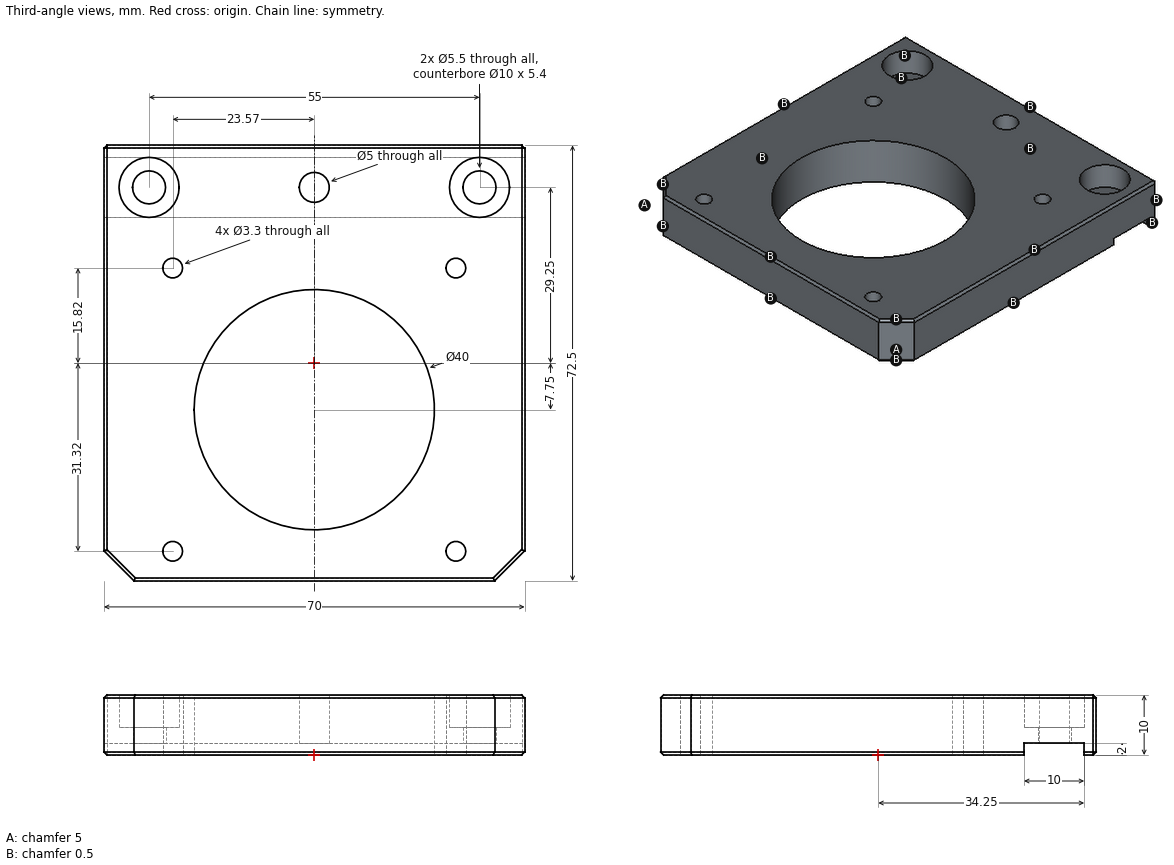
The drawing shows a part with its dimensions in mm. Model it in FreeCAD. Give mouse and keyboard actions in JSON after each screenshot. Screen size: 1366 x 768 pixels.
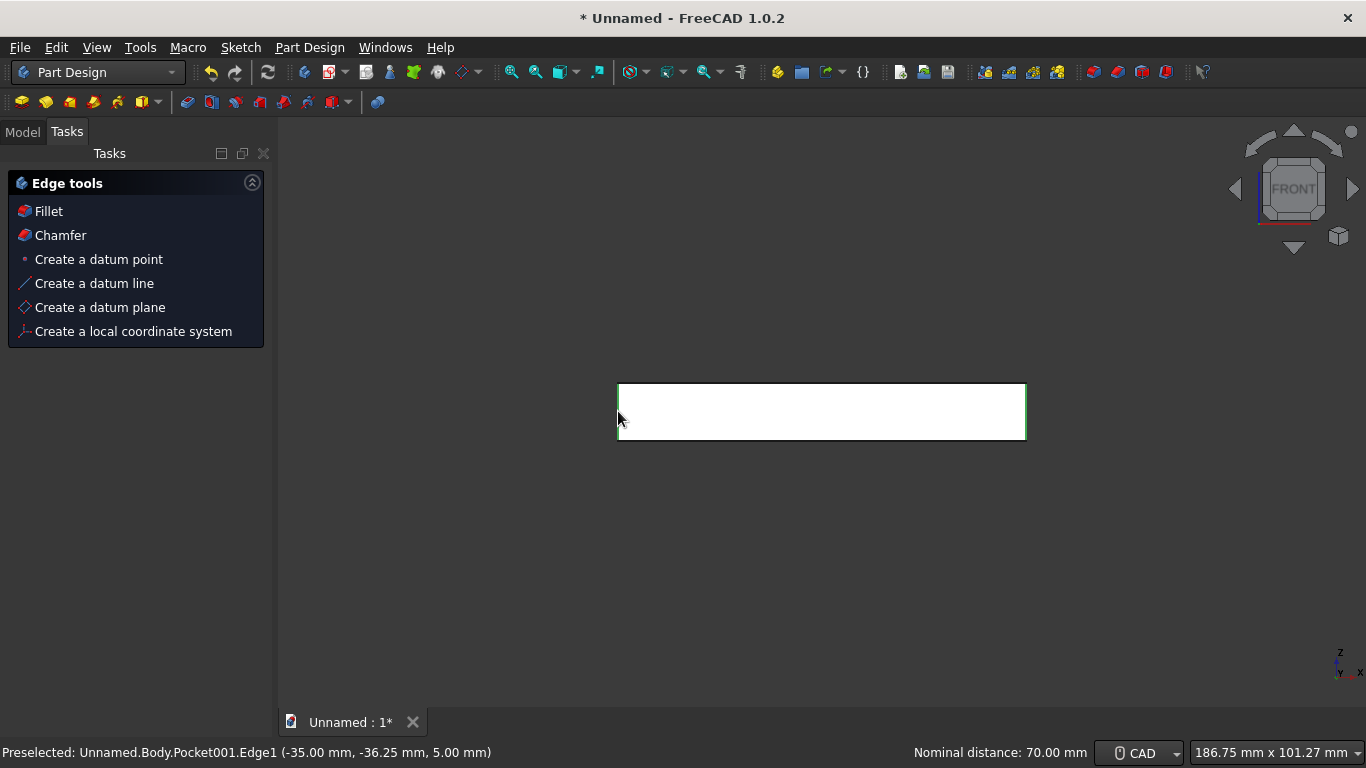
{"action": "left_click", "coordinate": [1118, 72]}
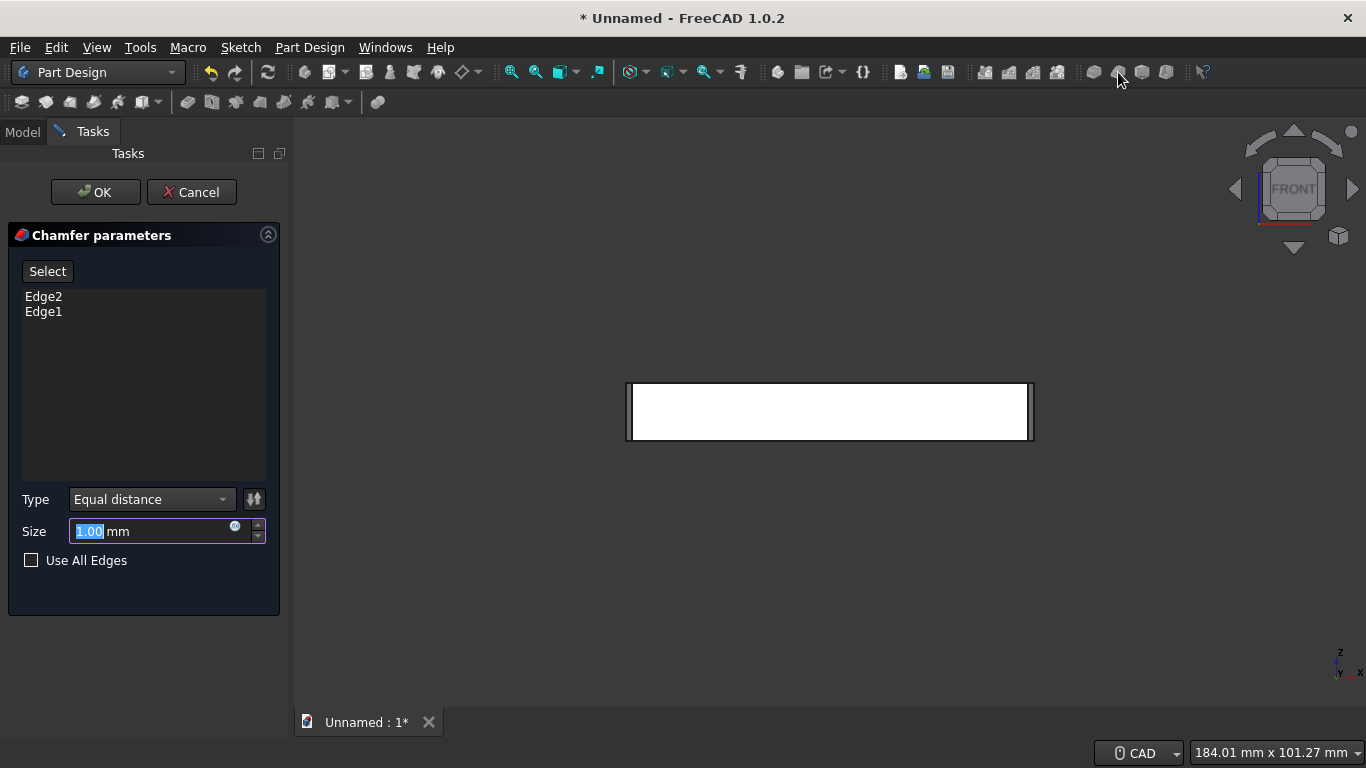
{"action": "type", "text": "5"}
{"action": "key", "text": "Tab"}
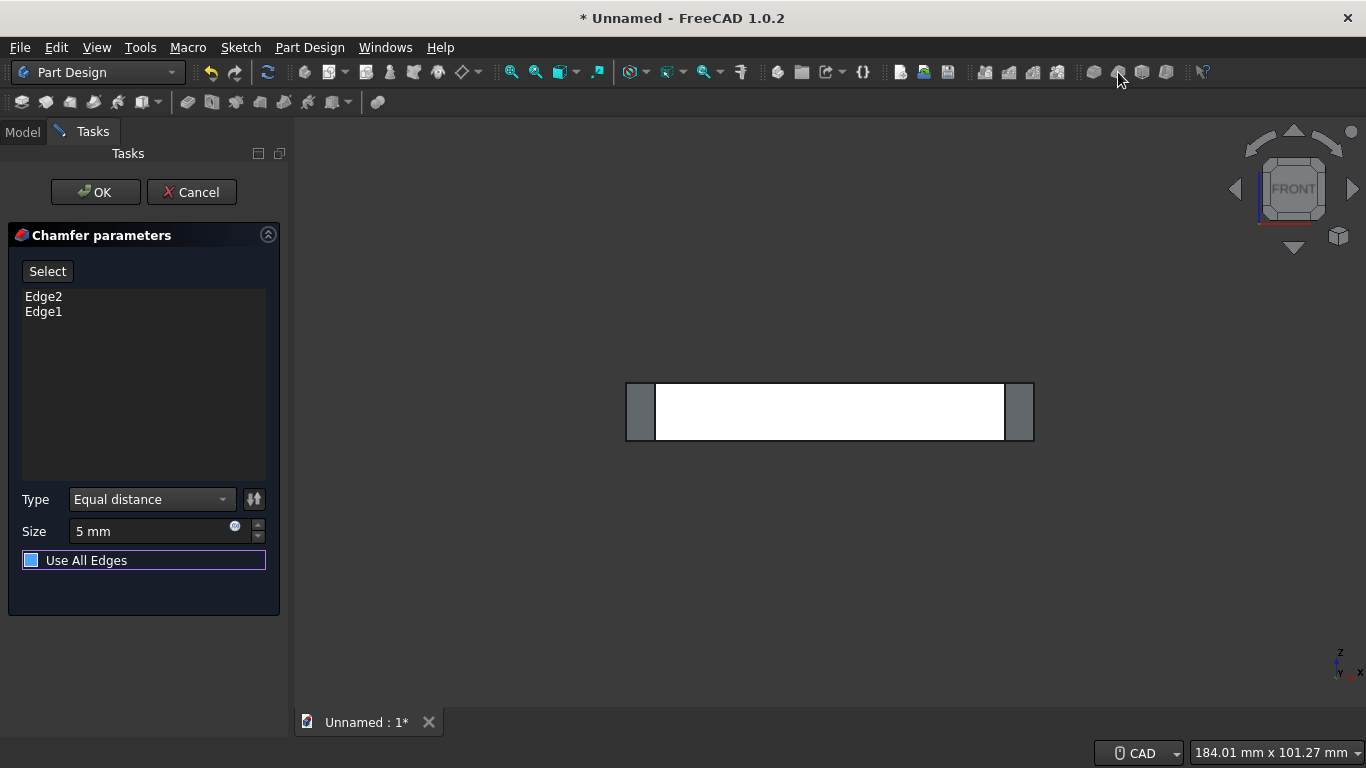
{"action": "left_click", "coordinate": [96, 192]}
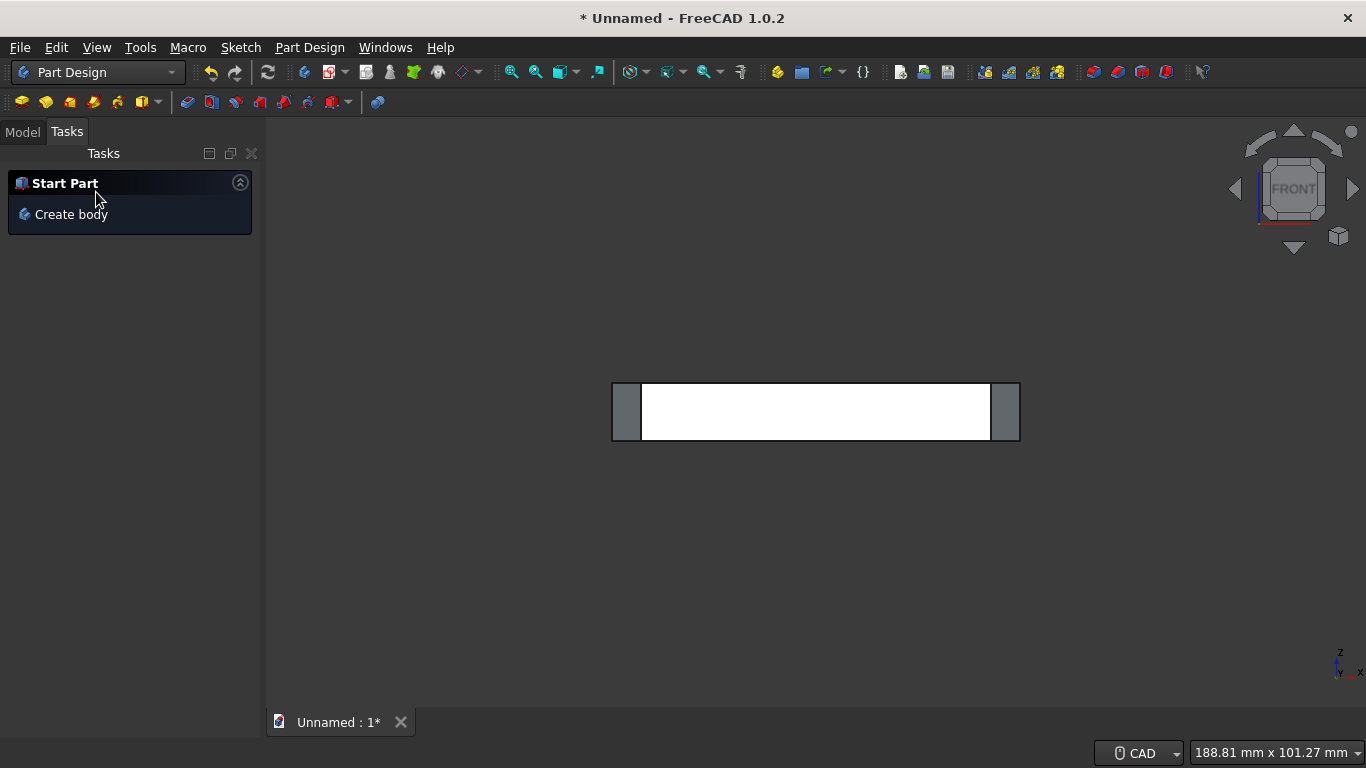
{"action": "left_click", "coordinate": [512, 72]}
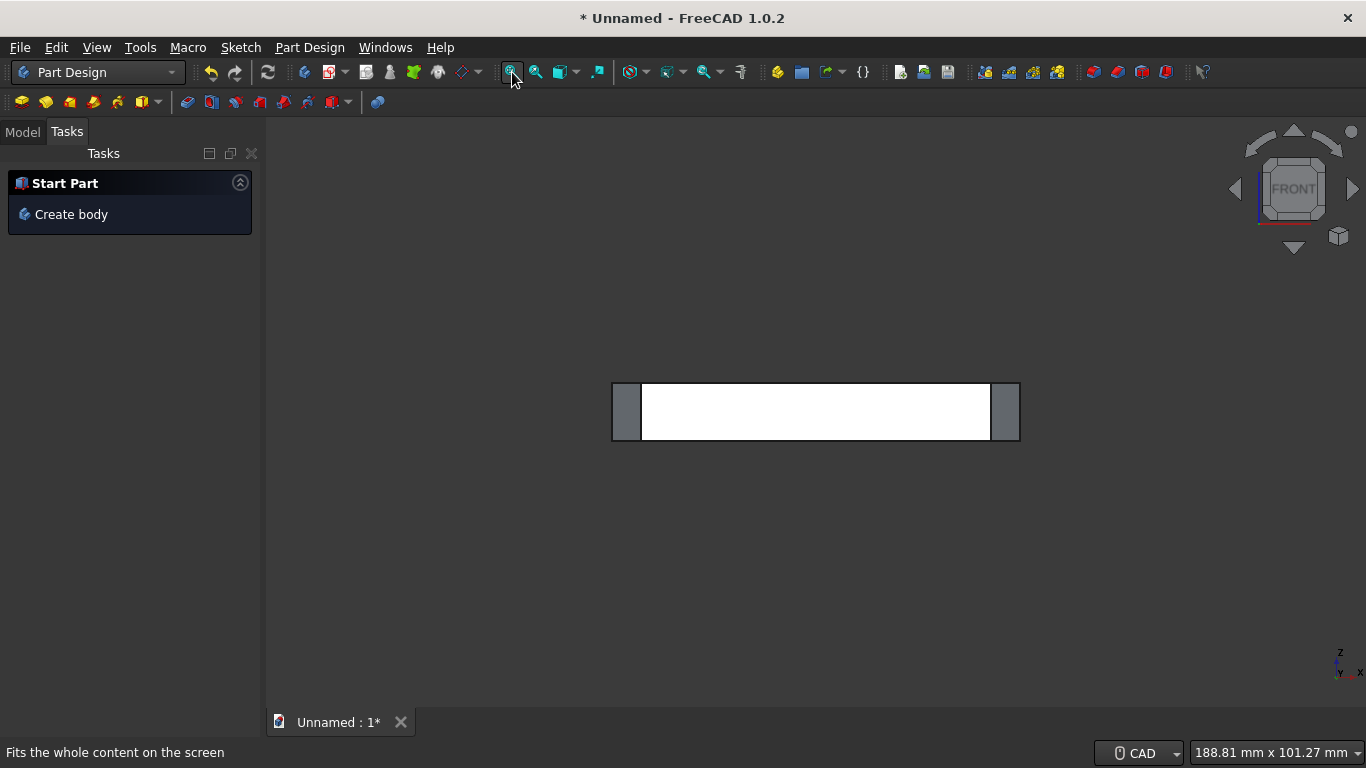
{"action": "left_click", "coordinate": [816, 440]}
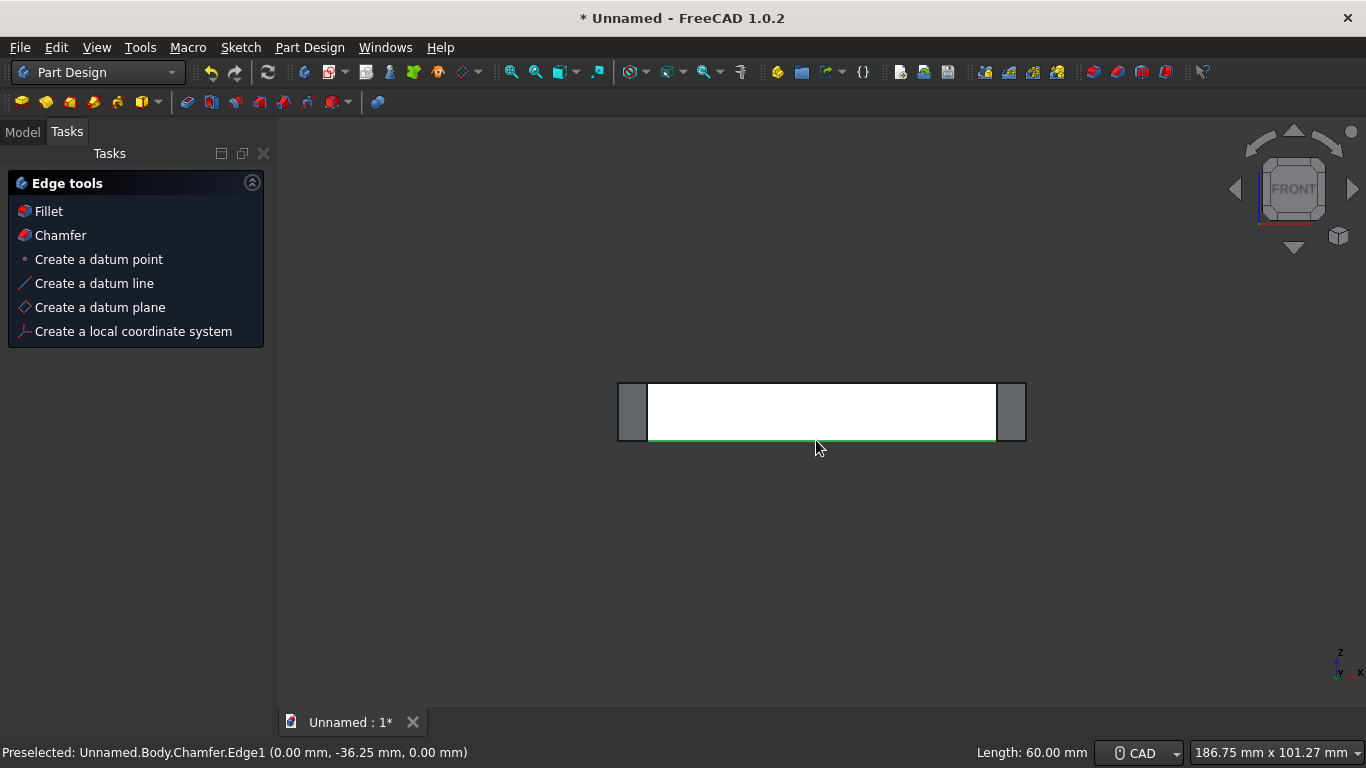
{"action": "left_click", "coordinate": [633, 440], "text": "ctrl"}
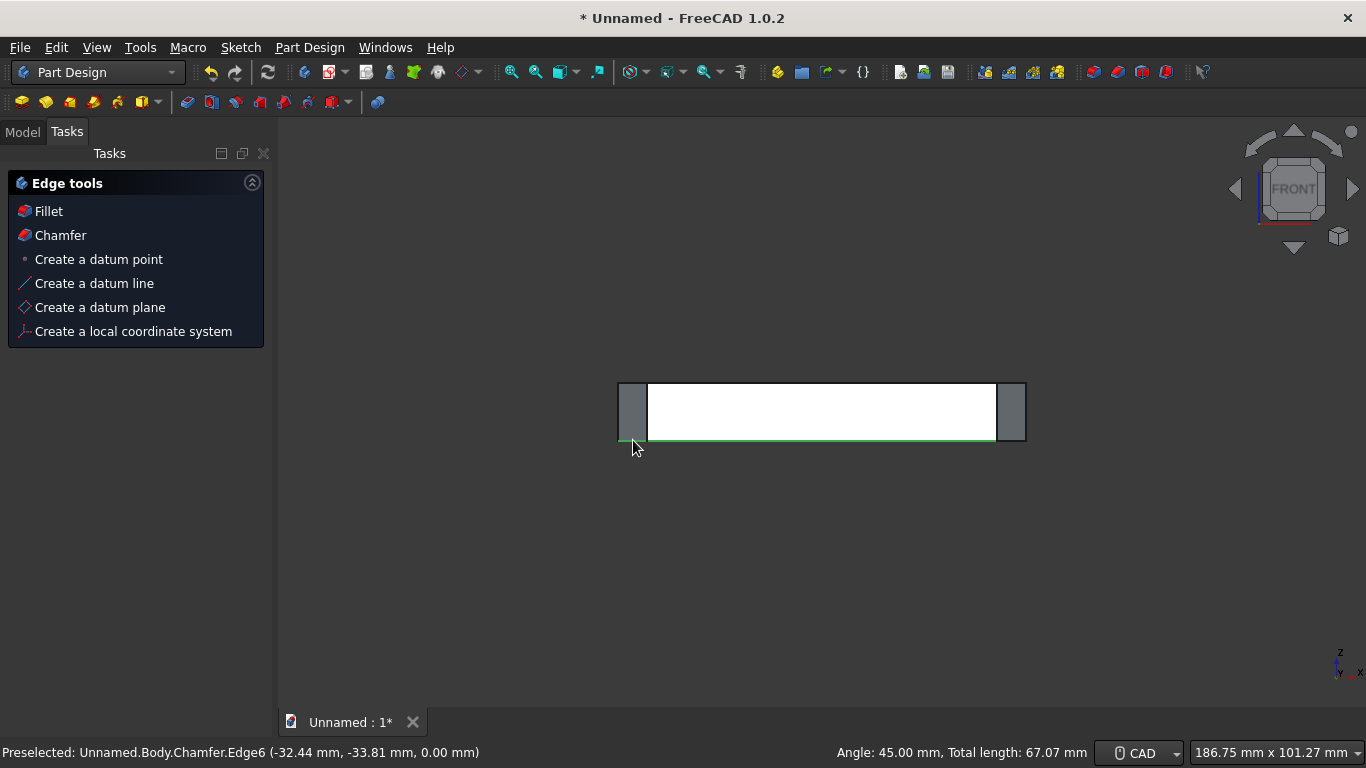
{"action": "left_click", "coordinate": [1011, 440], "text": "ctrl"}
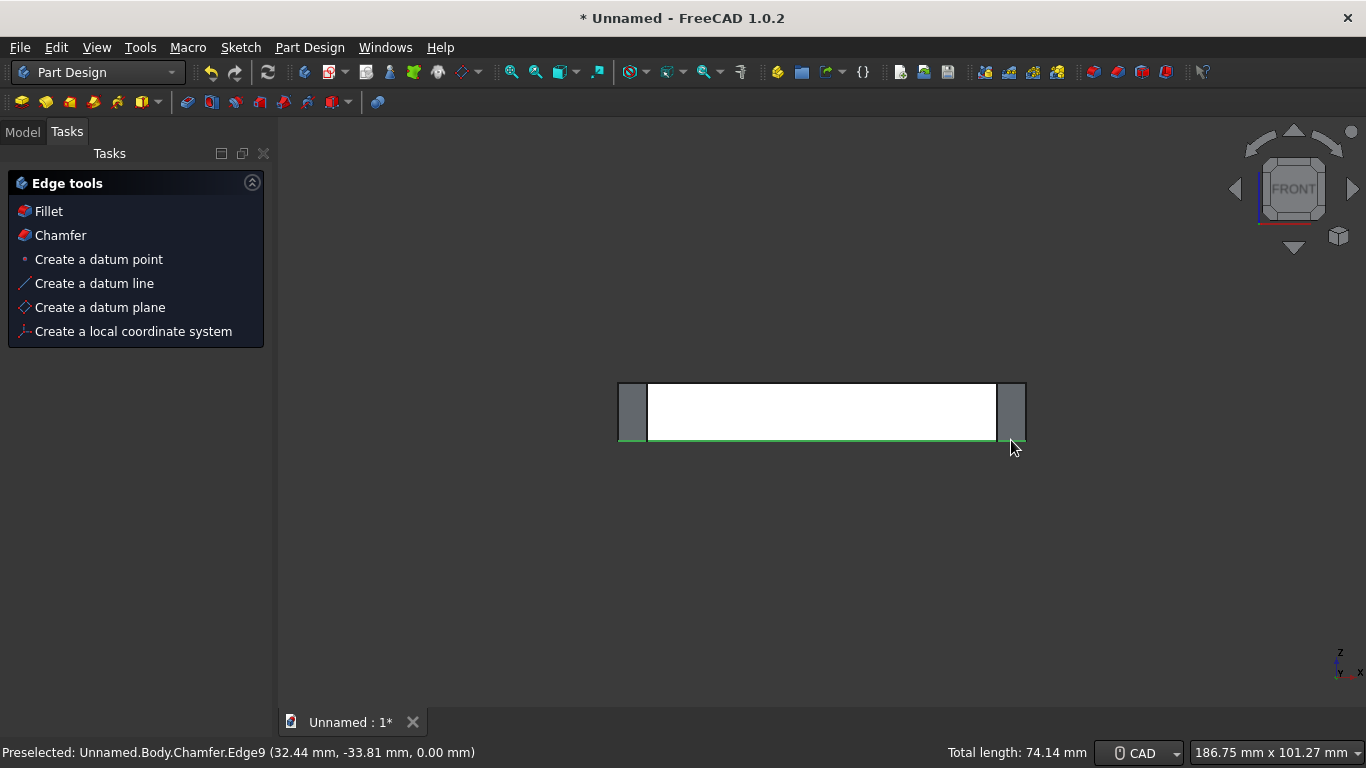
{"action": "left_click", "coordinate": [822, 382], "text": "ctrl"}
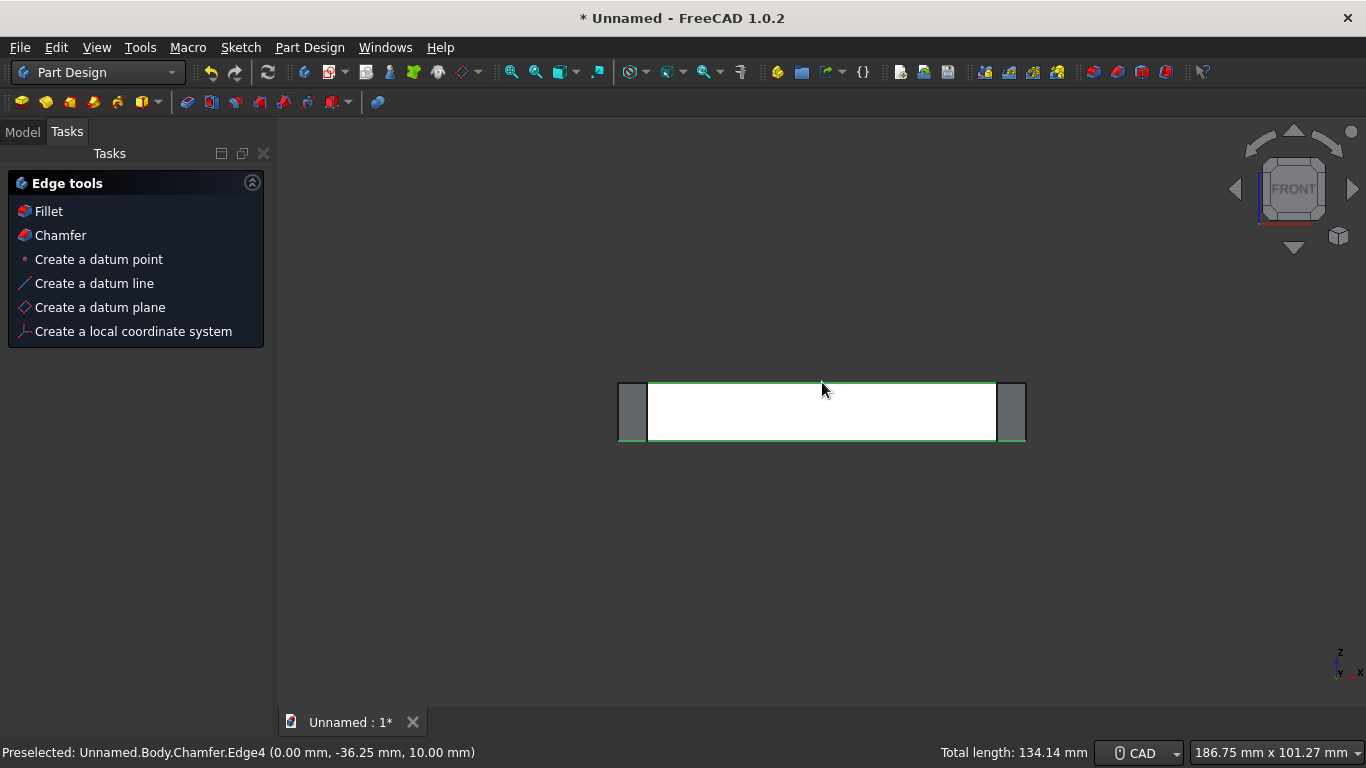
{"action": "left_click", "coordinate": [633, 382], "text": "ctrl"}